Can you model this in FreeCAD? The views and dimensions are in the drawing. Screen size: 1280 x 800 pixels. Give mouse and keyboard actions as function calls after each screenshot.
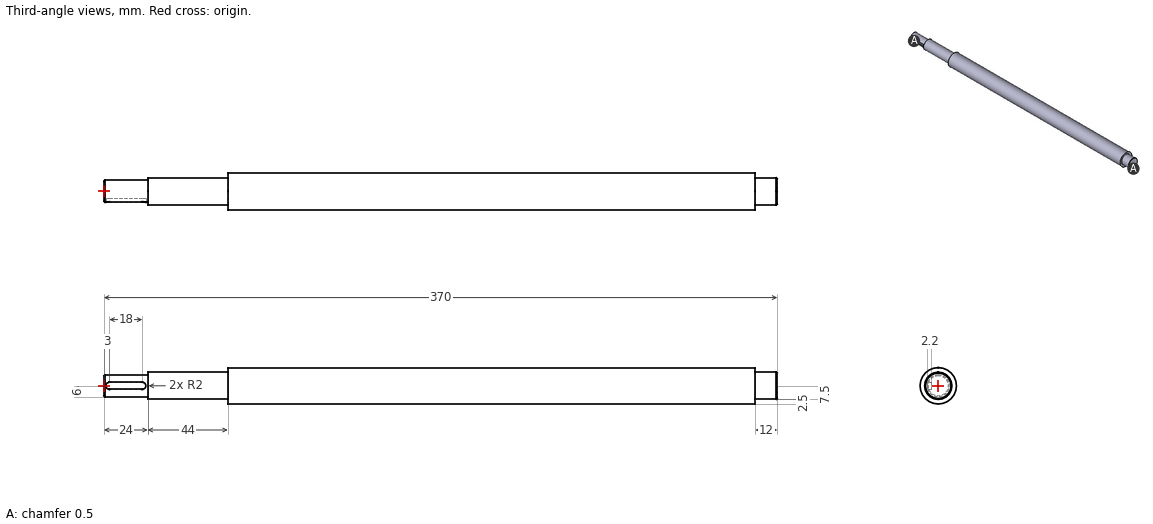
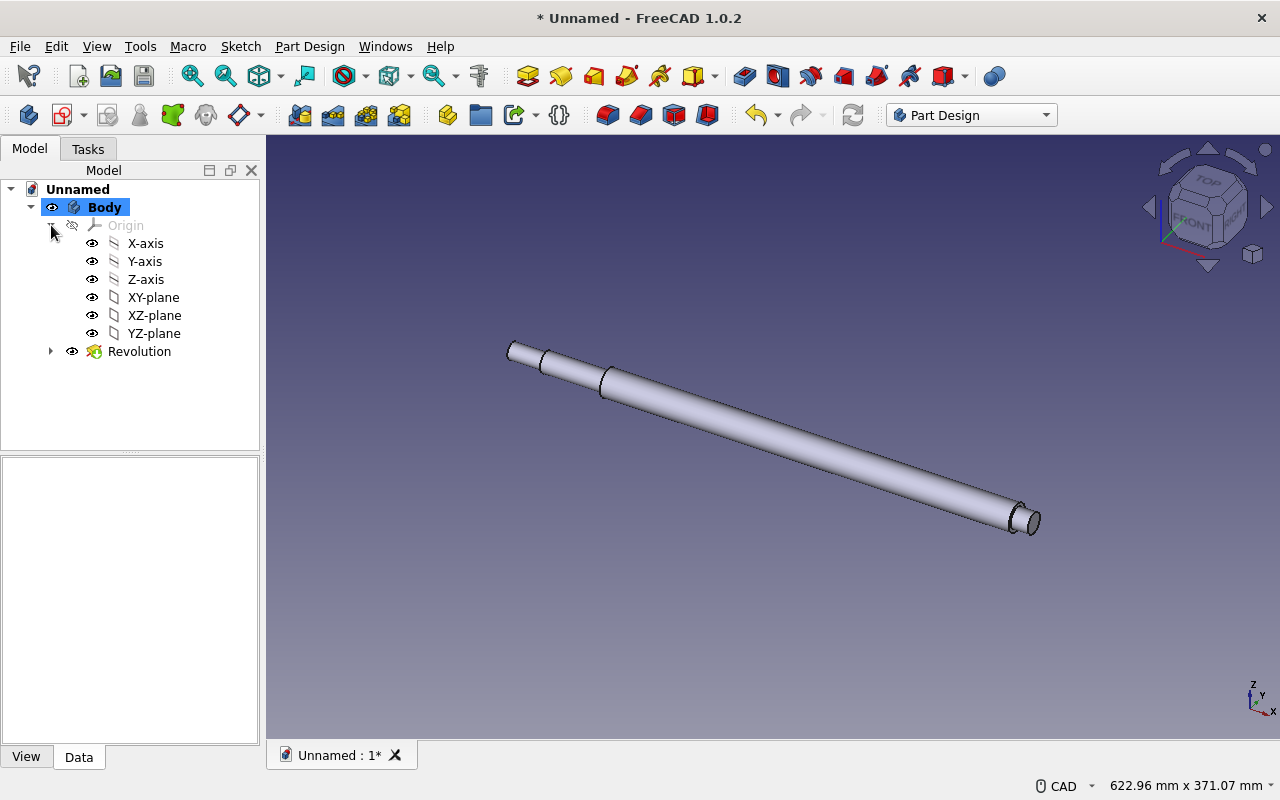
click(137, 315)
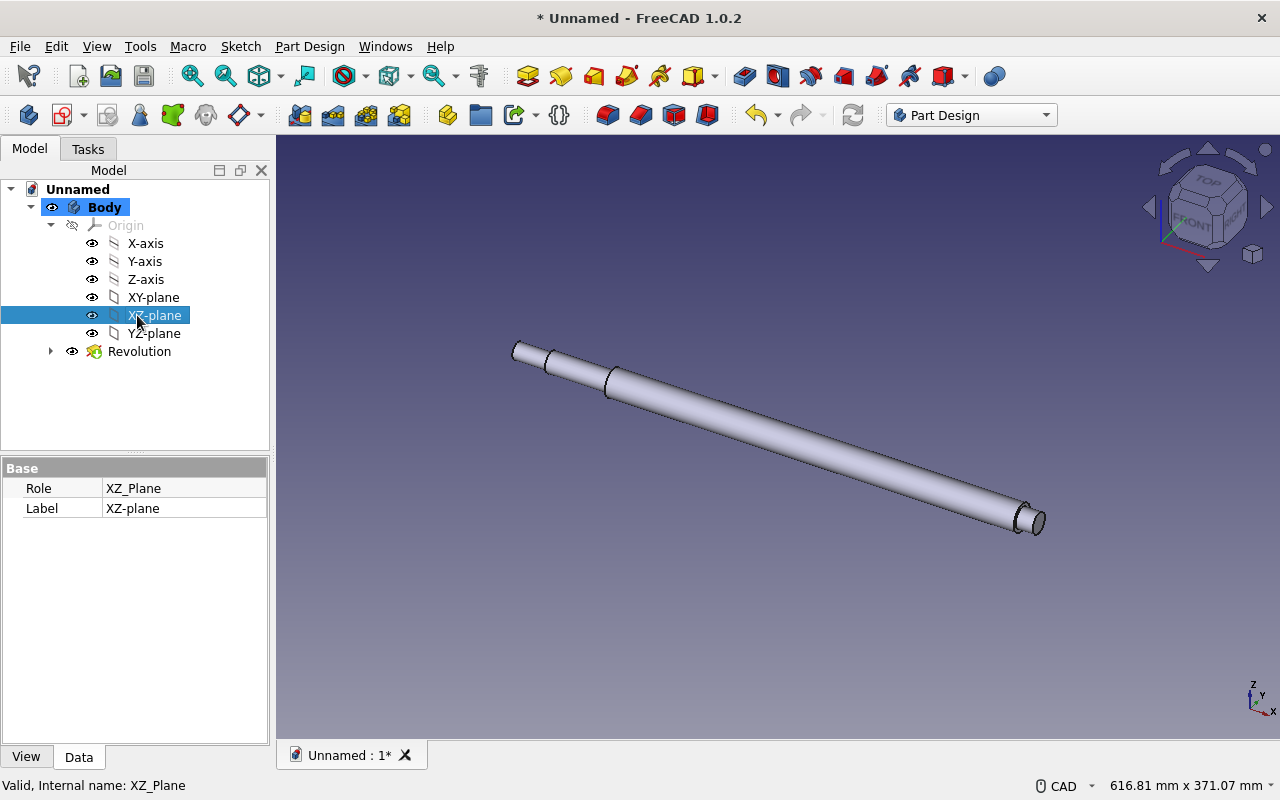
click(238, 116)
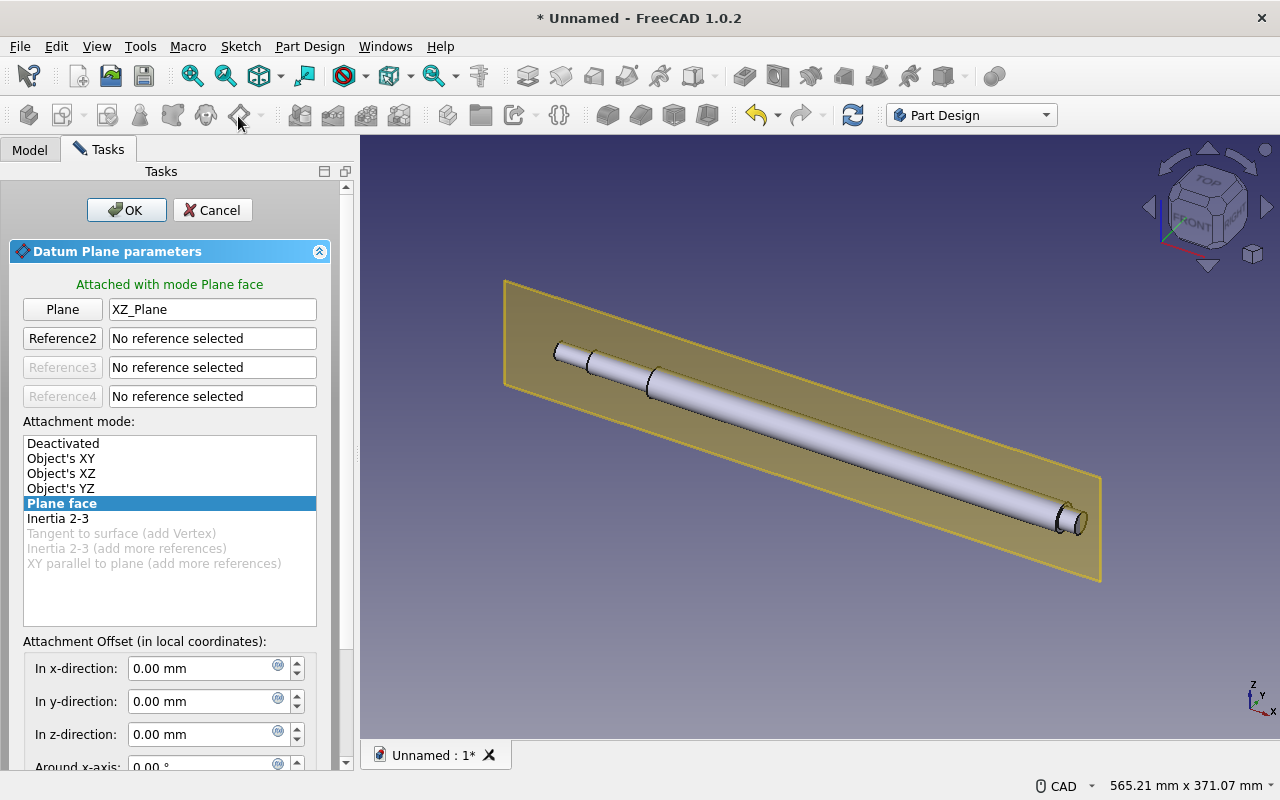
triple_click(210, 734)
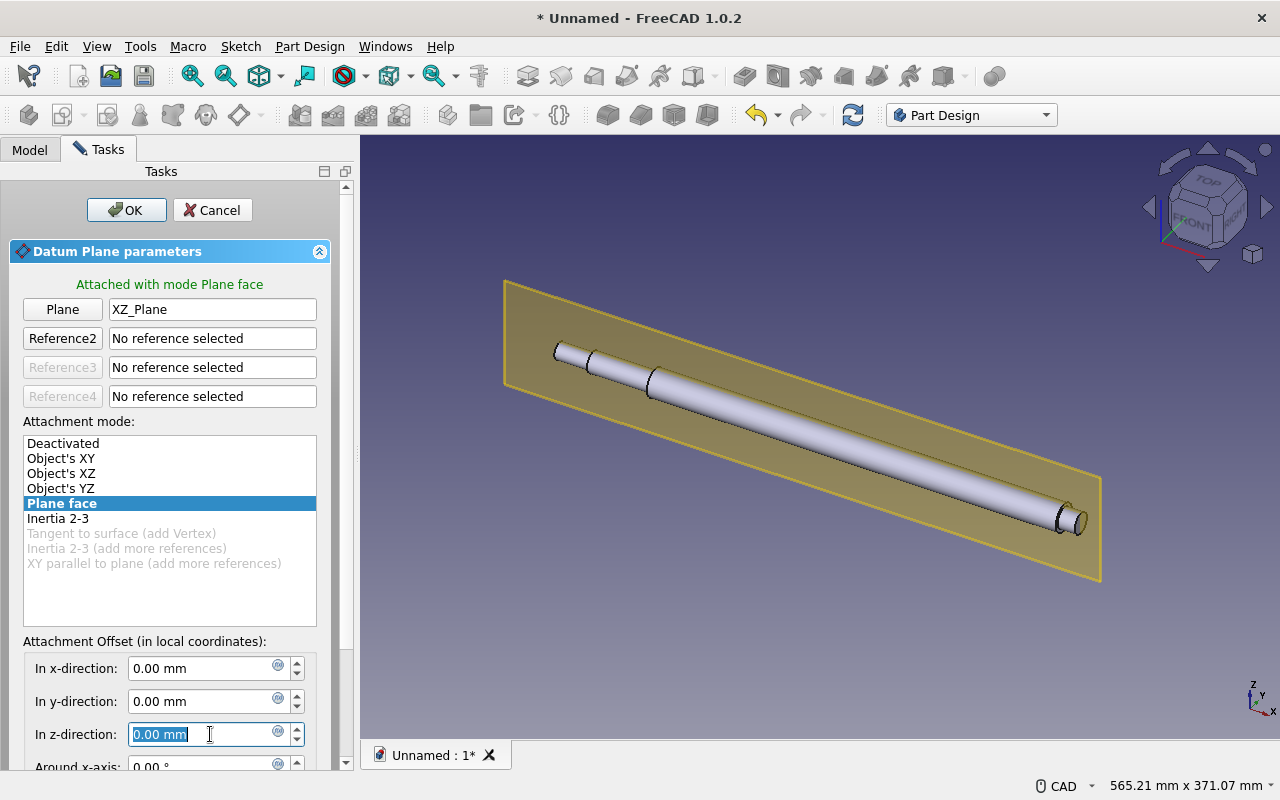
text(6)
key(Tab)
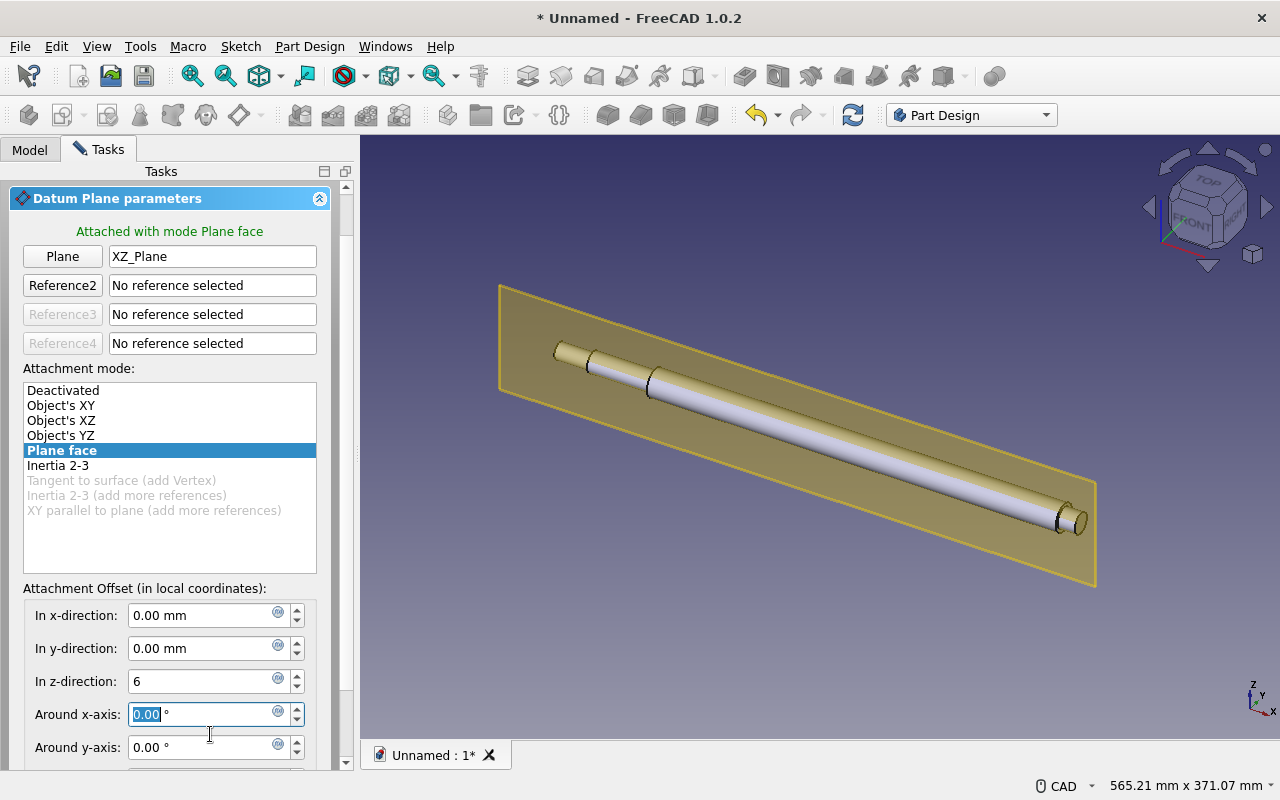
scroll(346, 476, up, 2)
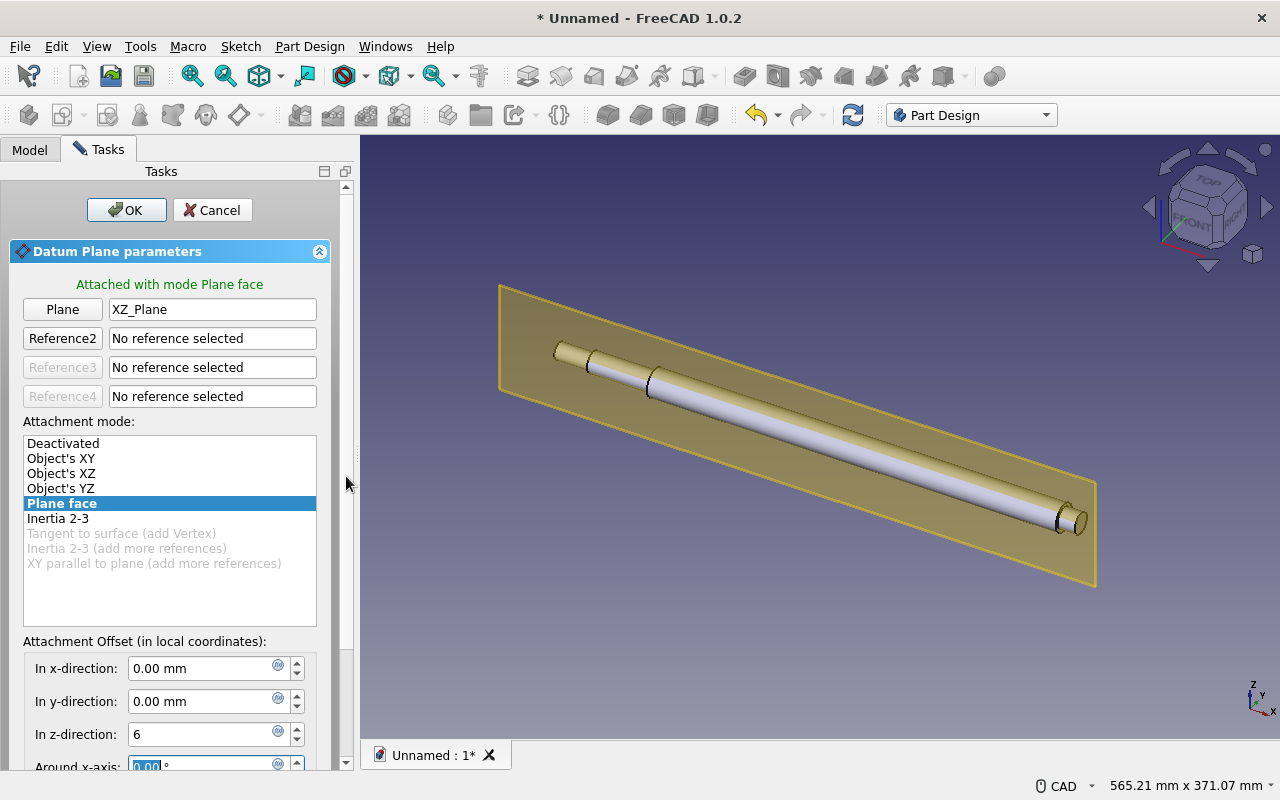
click(127, 210)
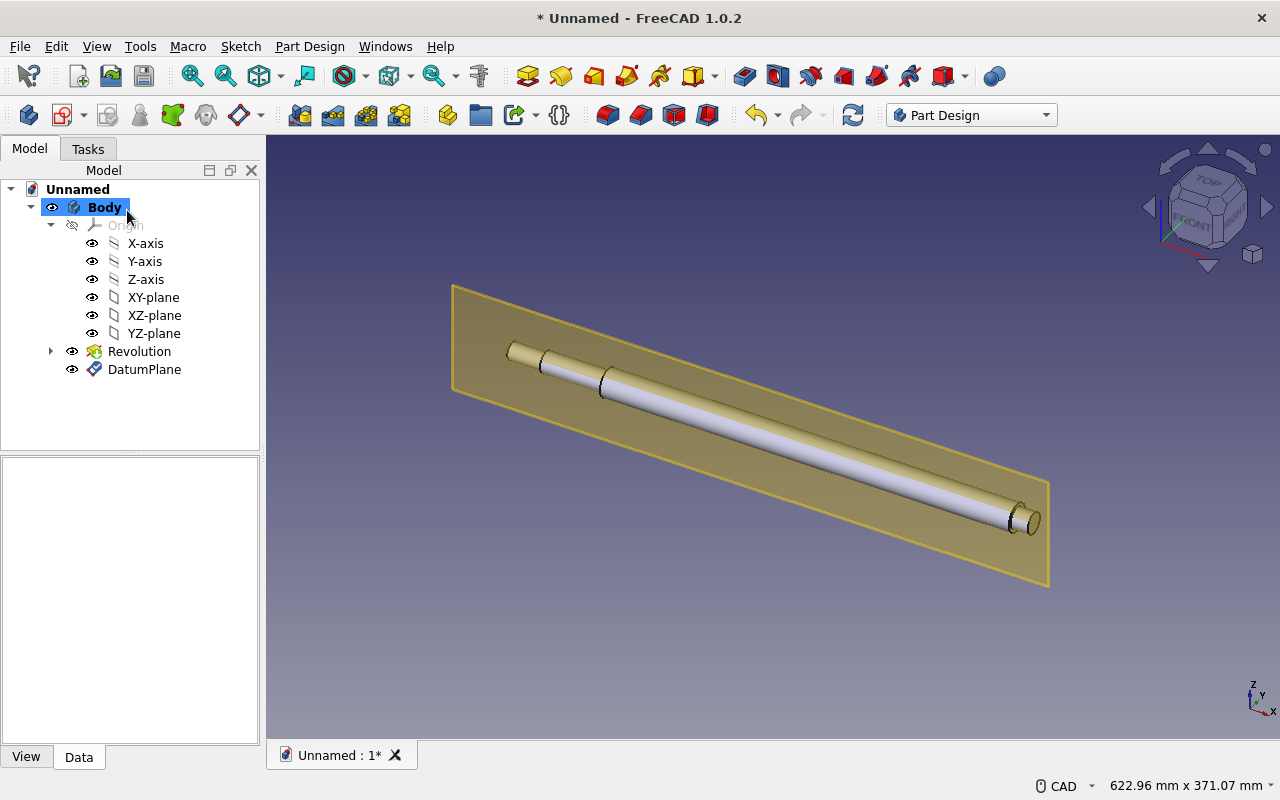
click(117, 369)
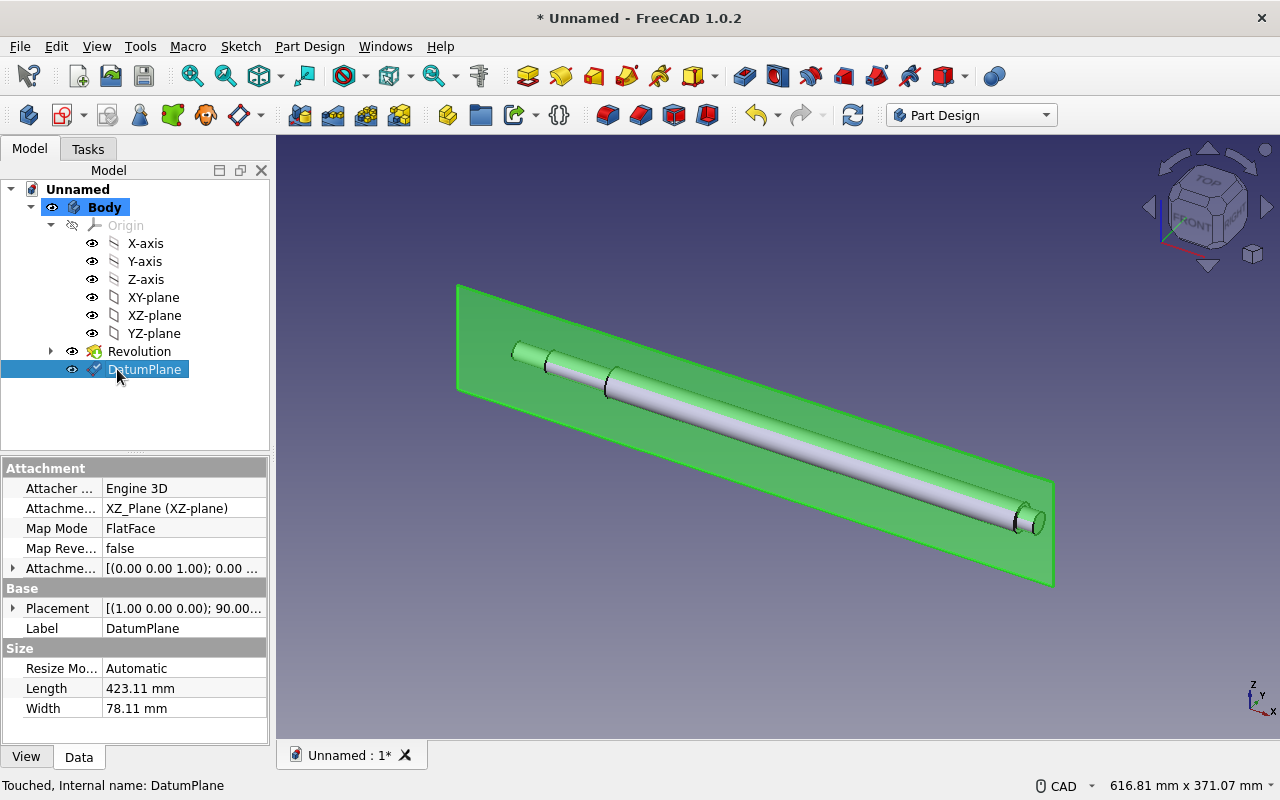
click(62, 116)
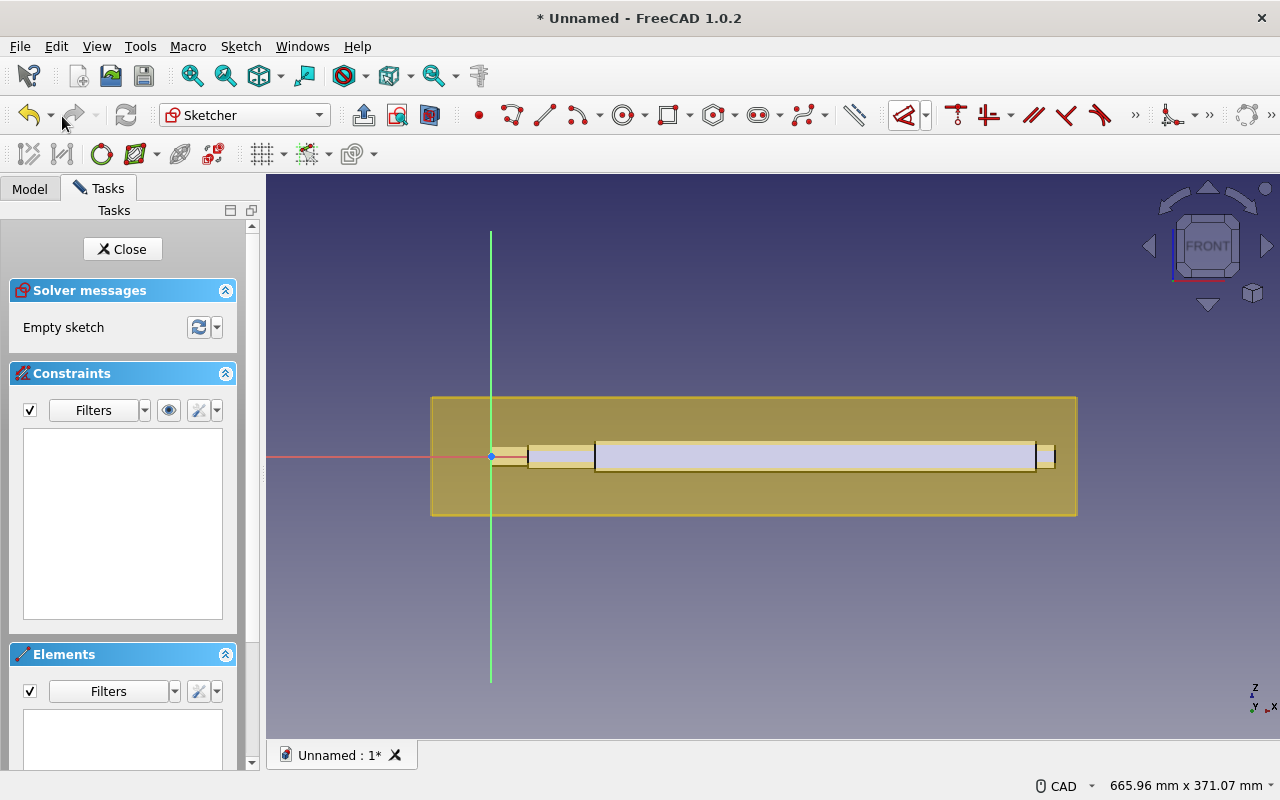
key(q)
key(s)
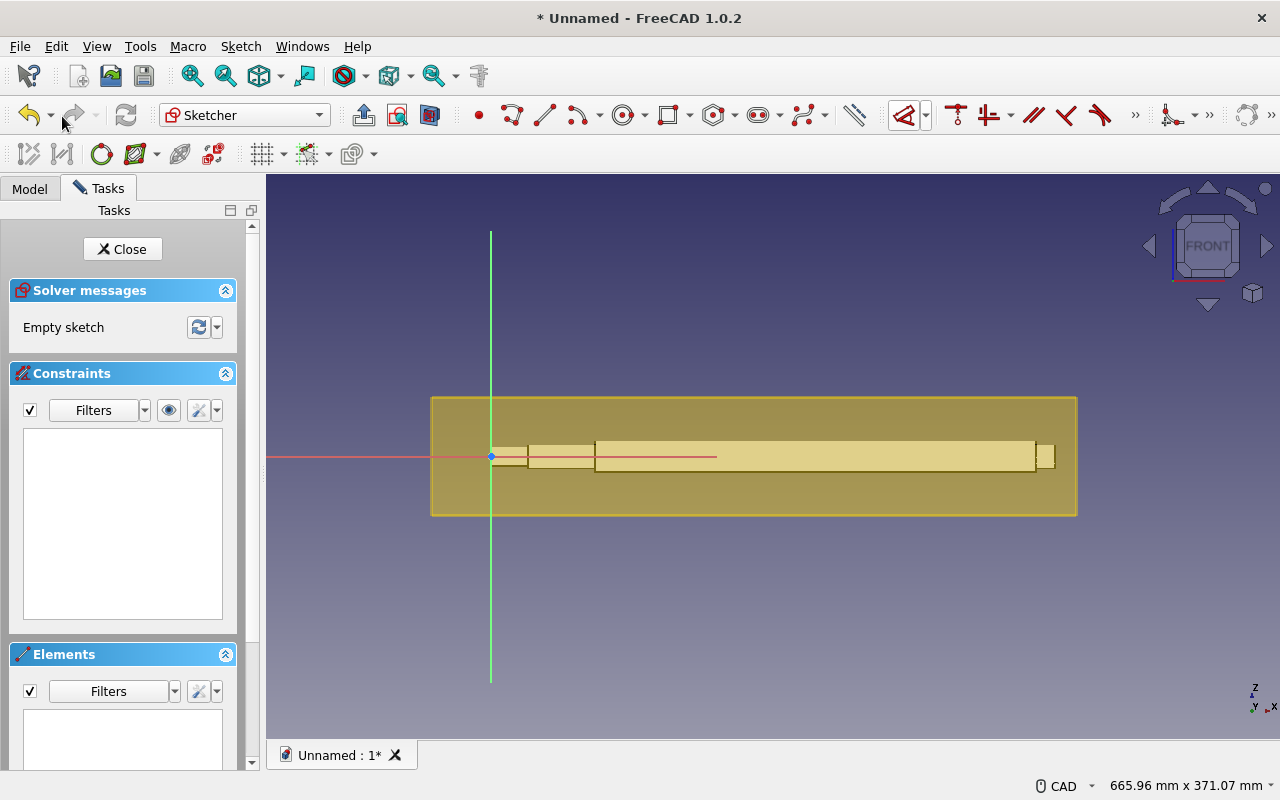
scroll(496, 457, up, 14)